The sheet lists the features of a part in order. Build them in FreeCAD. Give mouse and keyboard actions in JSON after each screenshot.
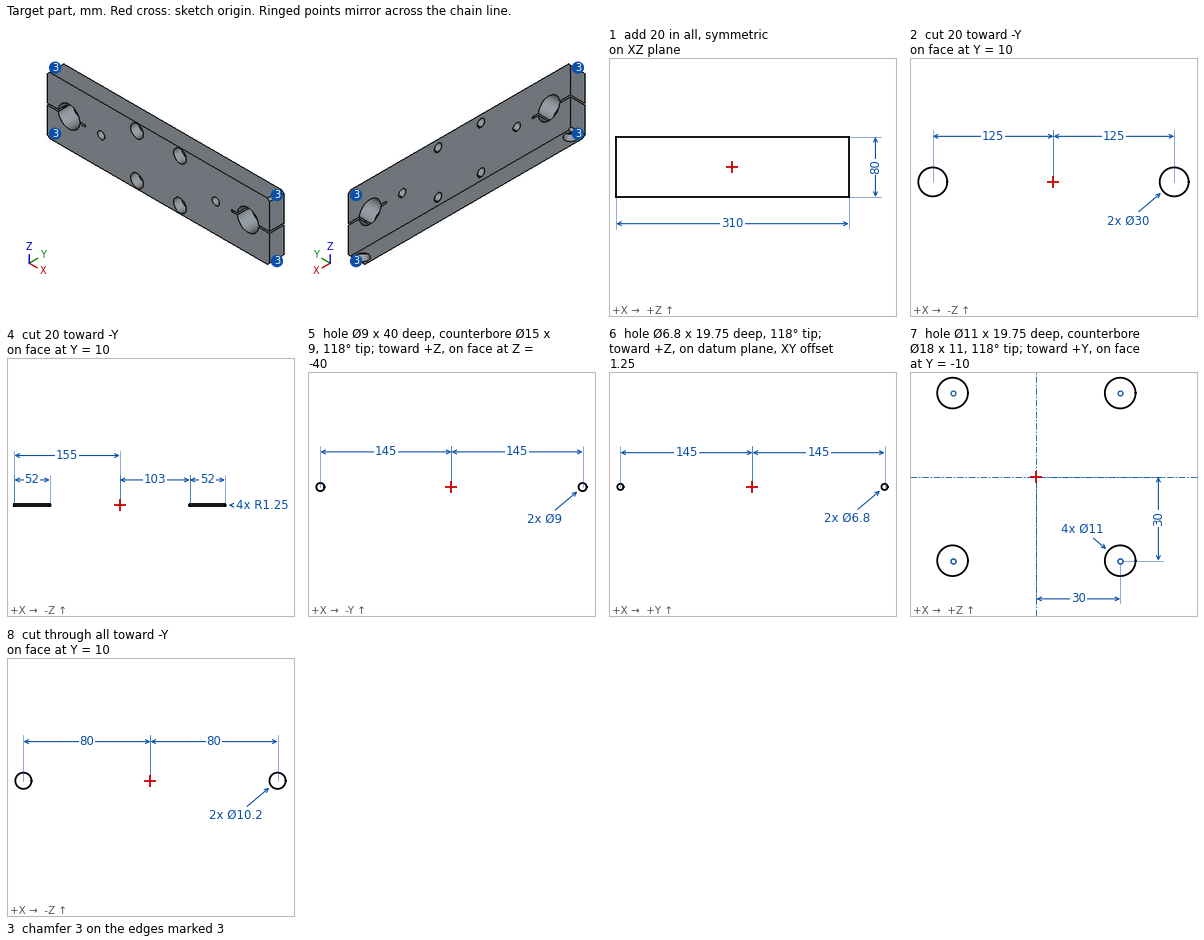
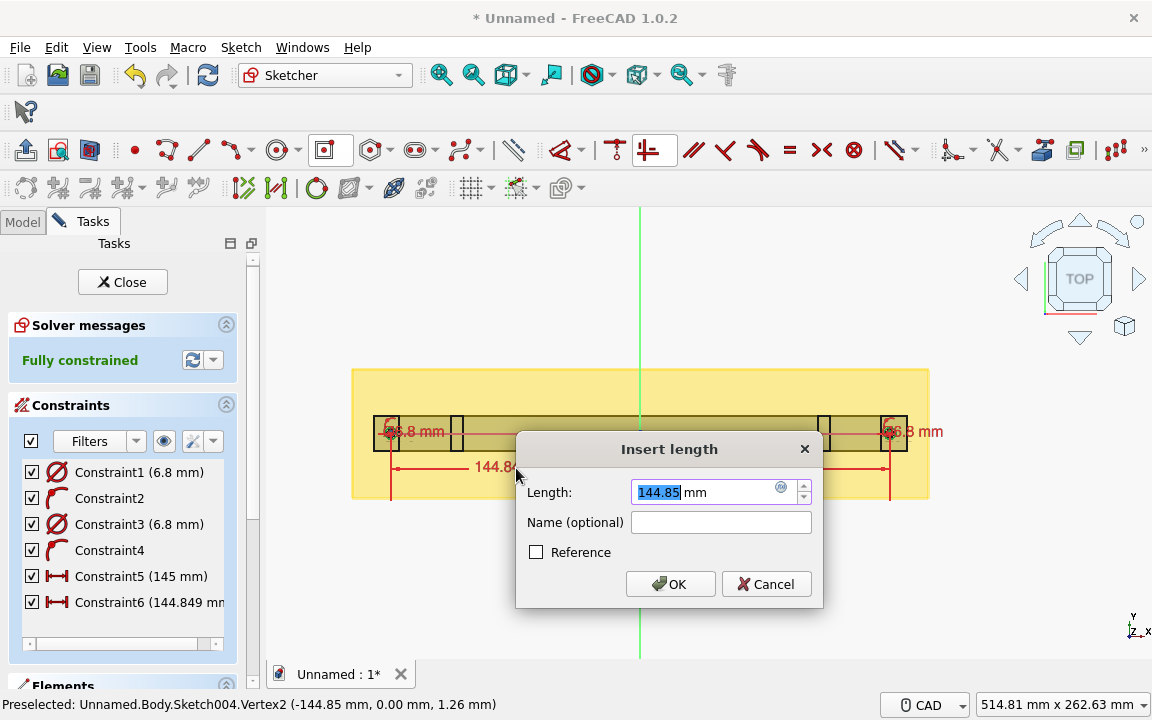
{"action": "type", "text": "145"}
{"action": "key", "text": "Return"}
{"action": "key", "text": "Escape"}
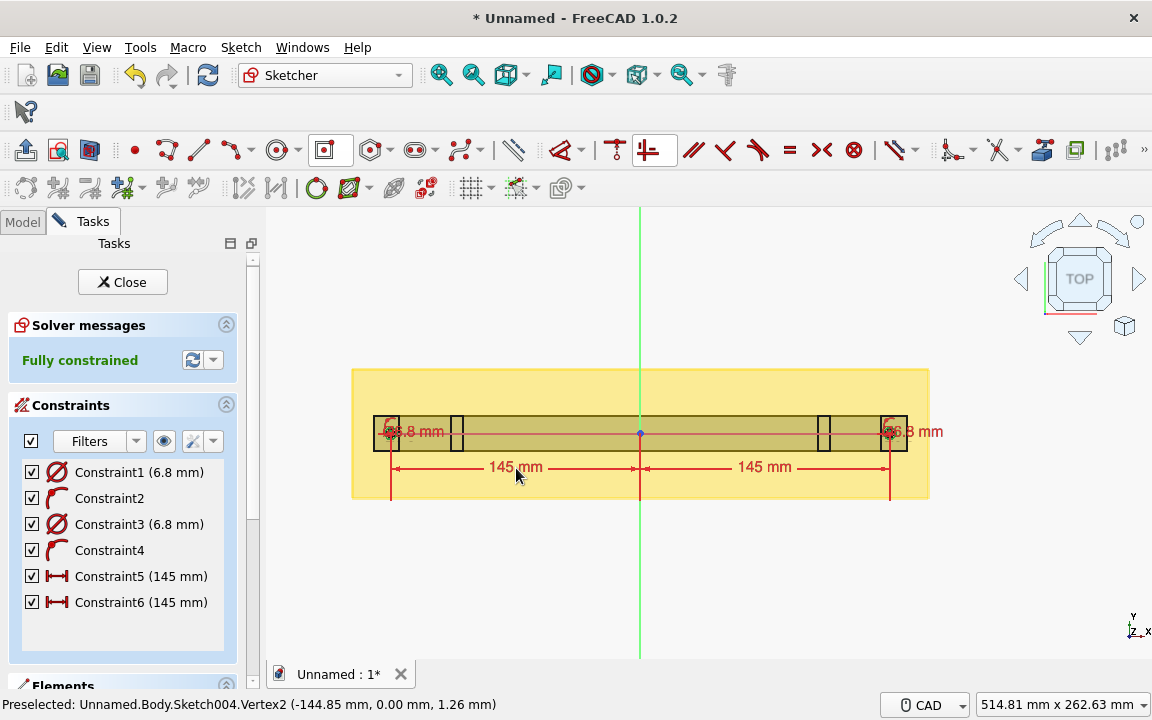
{"action": "left_click", "coordinate": [123, 282]}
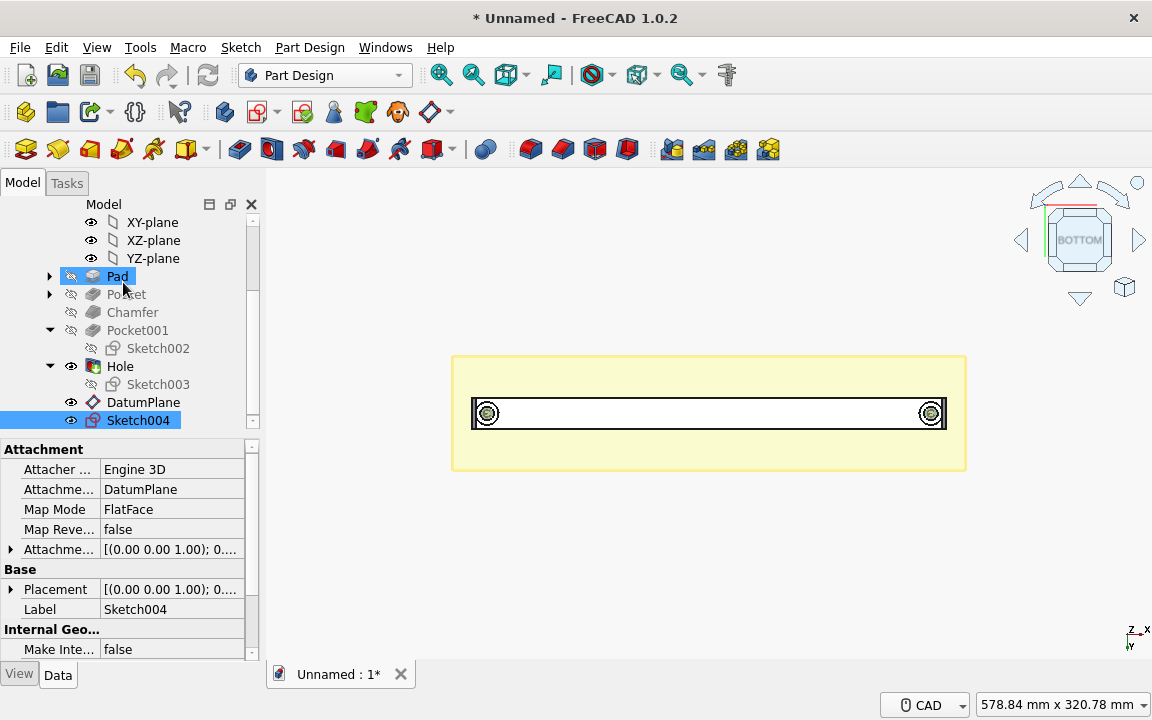
{"action": "left_click", "coordinate": [272, 150]}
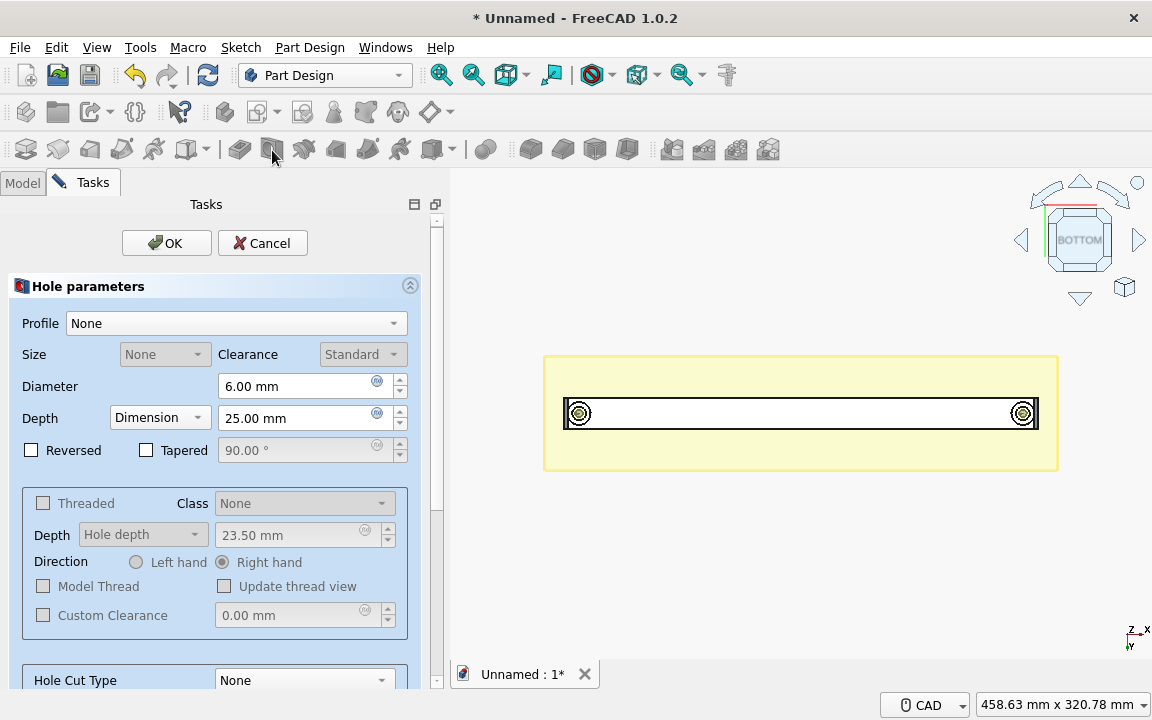
{"action": "triple_click", "coordinate": [305, 386]}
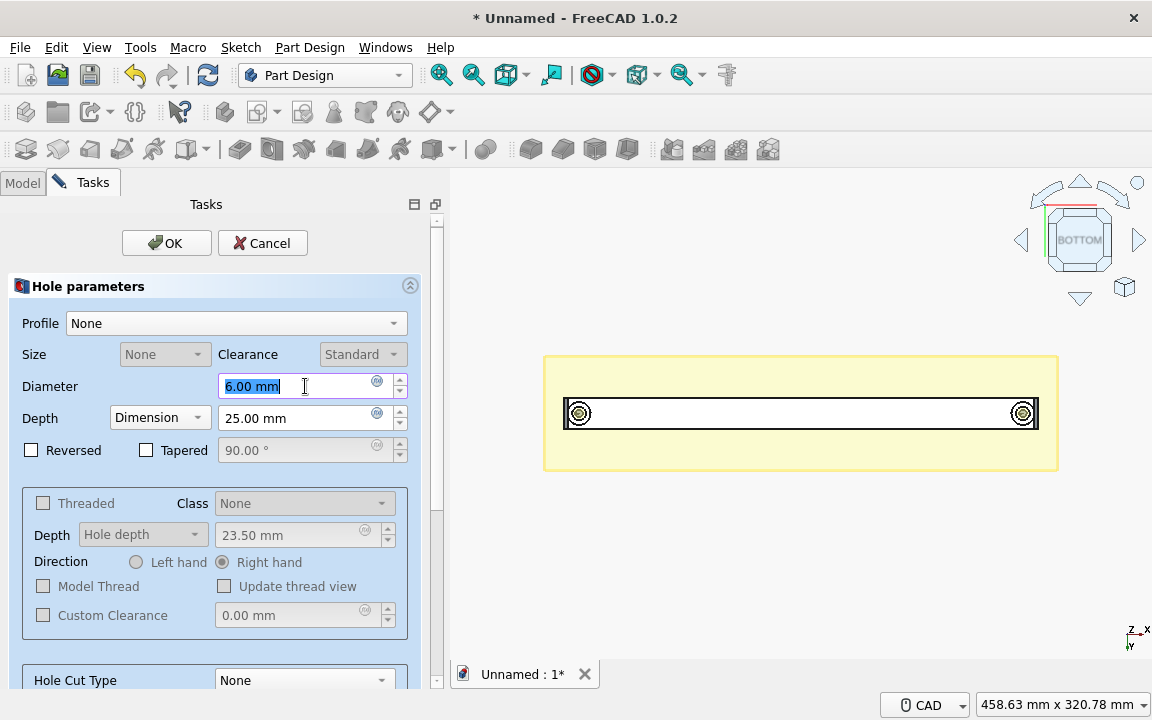
{"action": "type", "text": "6.8"}
{"action": "key", "text": "Tab"}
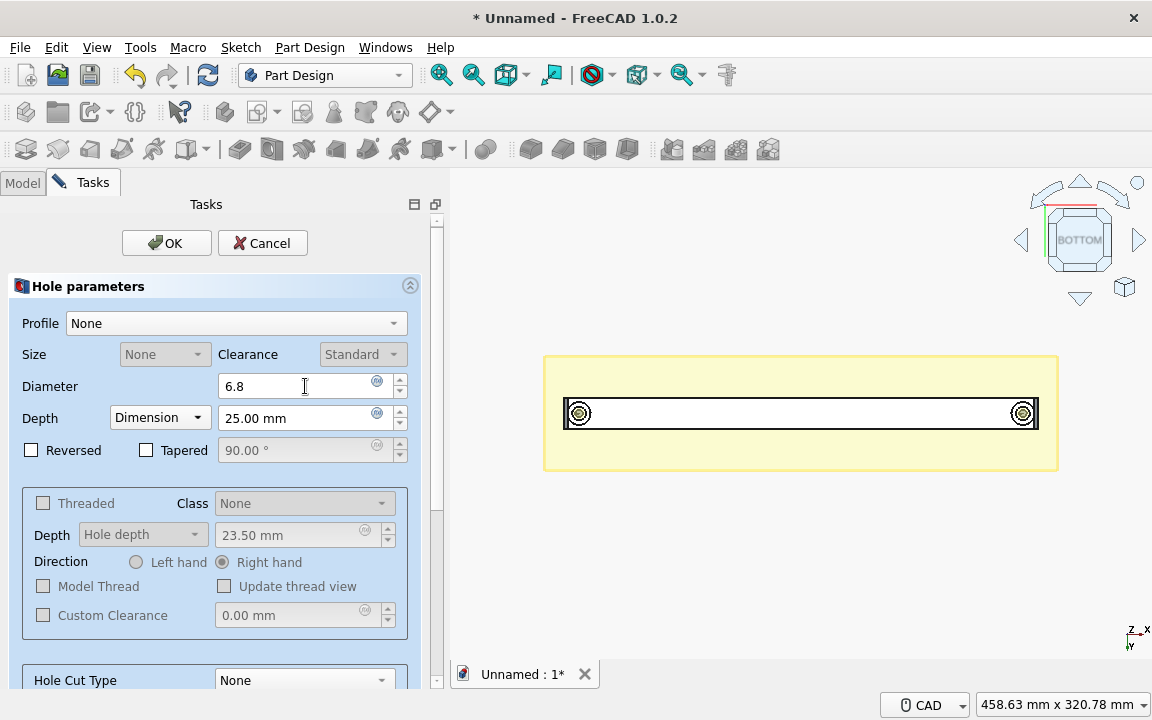
{"action": "triple_click", "coordinate": [305, 418]}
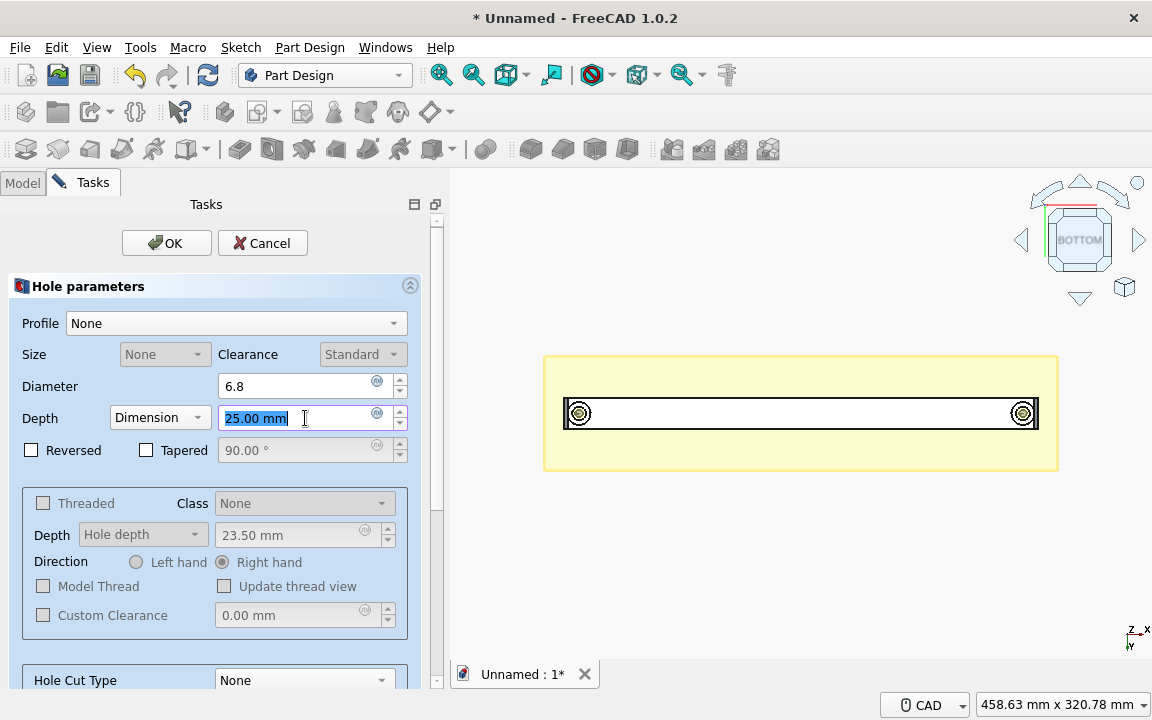
{"action": "type", "text": "19.75"}
{"action": "key", "text": "Tab"}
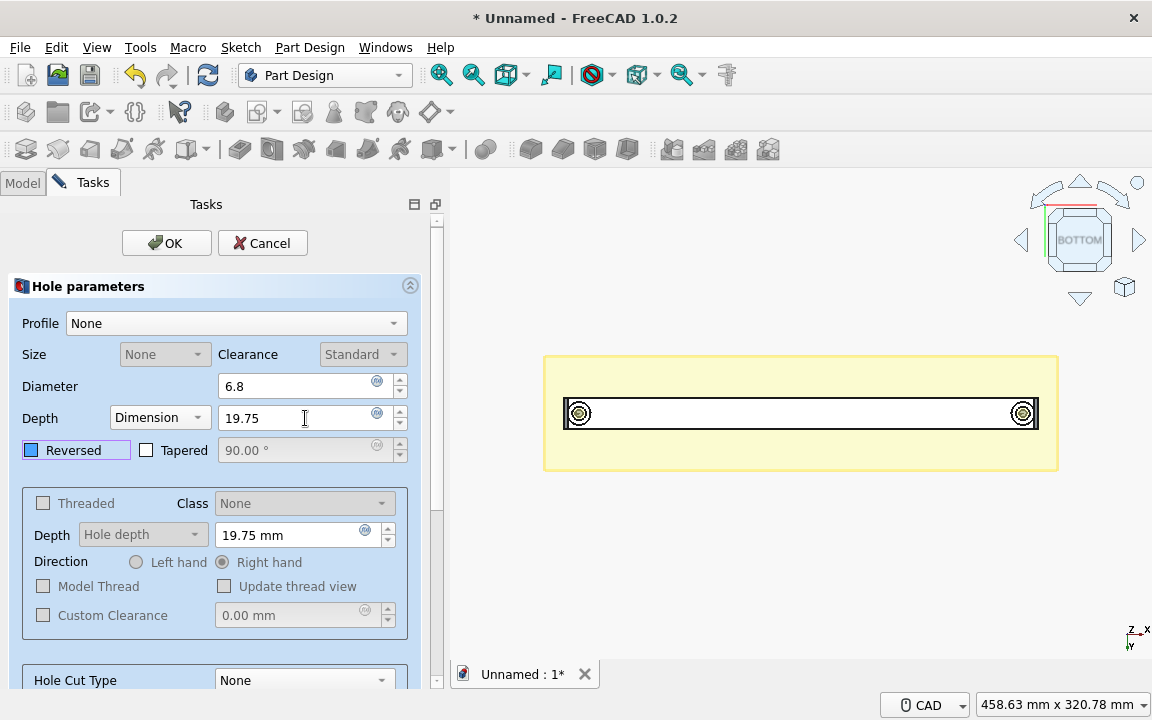
{"action": "left_click", "coordinate": [30, 450]}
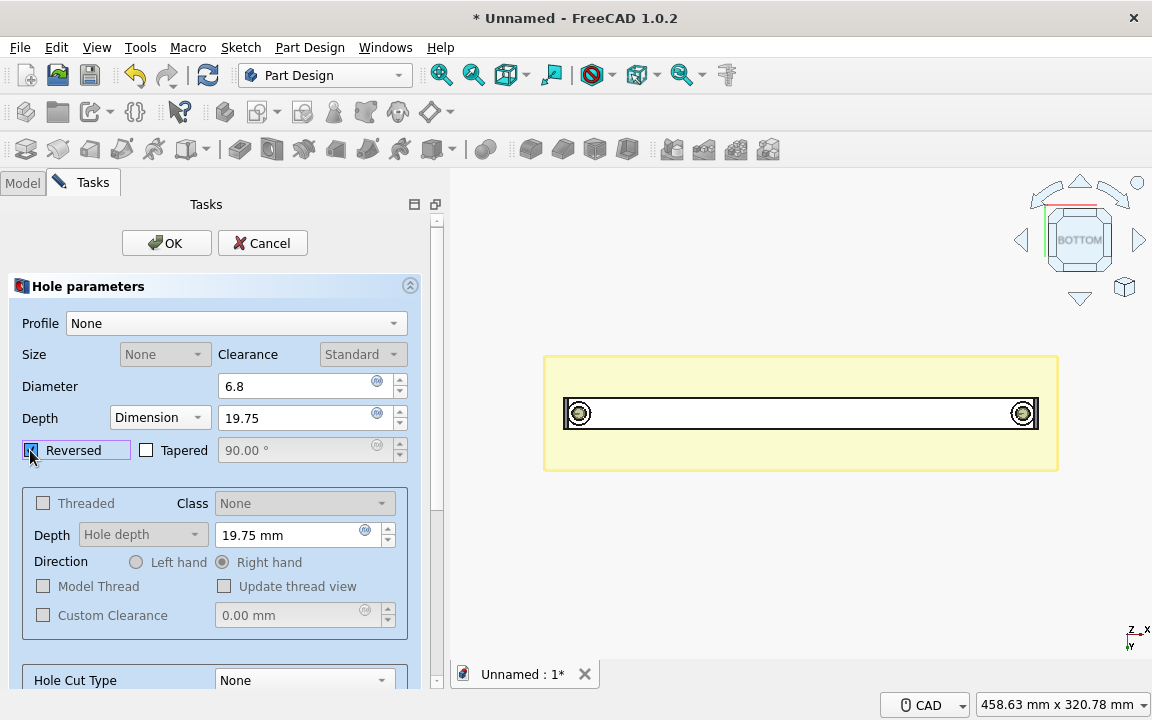
{"action": "left_click", "coordinate": [167, 243]}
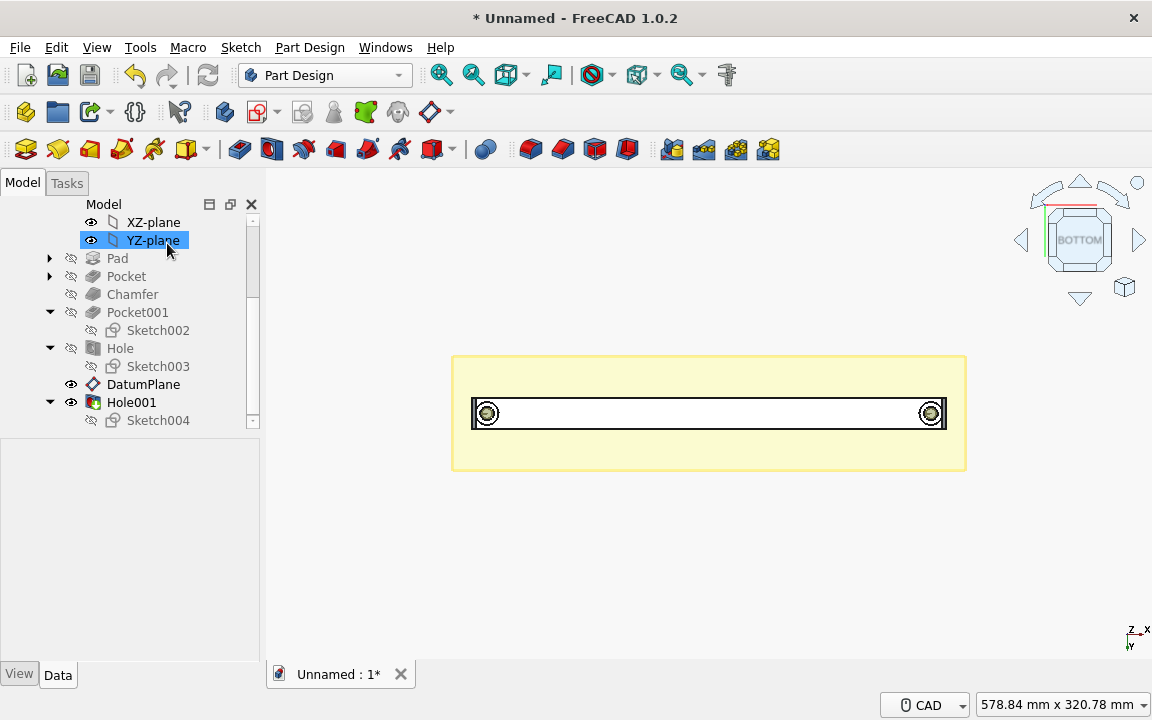
{"action": "left_click", "coordinate": [116, 384]}
{"action": "key", "text": "space"}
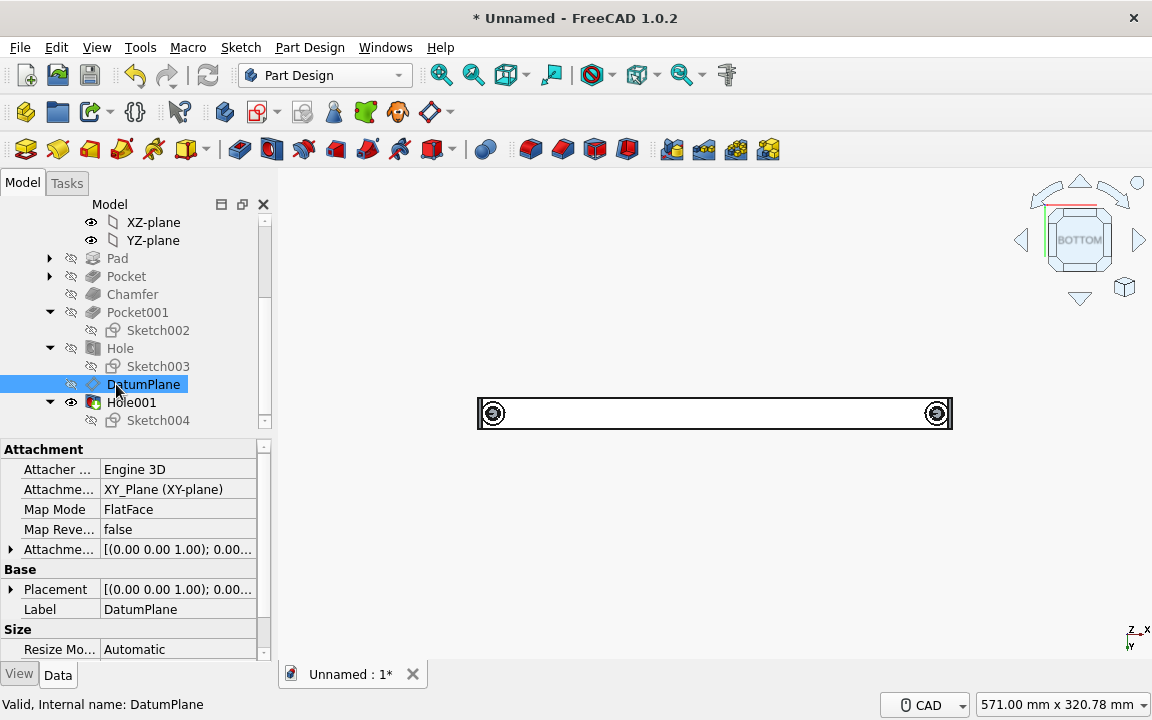
{"action": "key", "text": "0"}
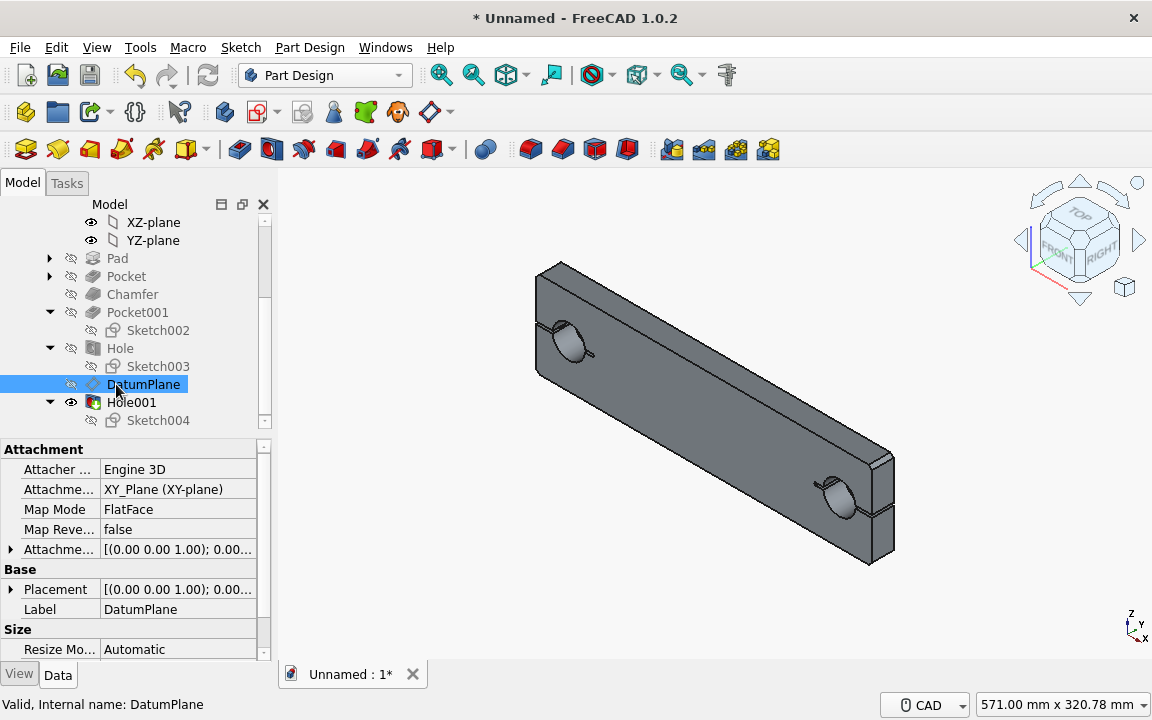
{"action": "left_click", "coordinate": [752, 446]}